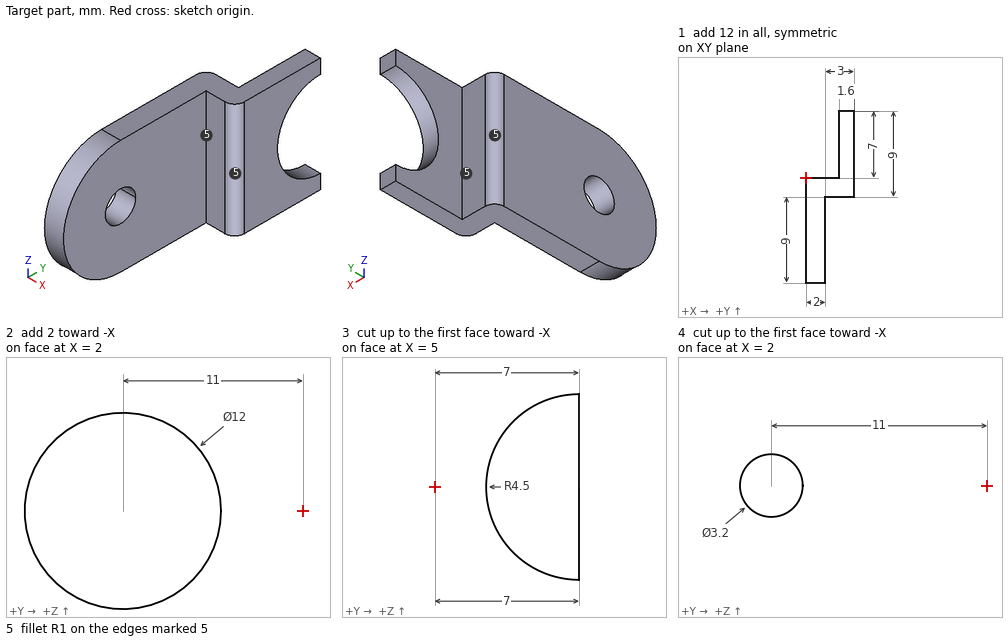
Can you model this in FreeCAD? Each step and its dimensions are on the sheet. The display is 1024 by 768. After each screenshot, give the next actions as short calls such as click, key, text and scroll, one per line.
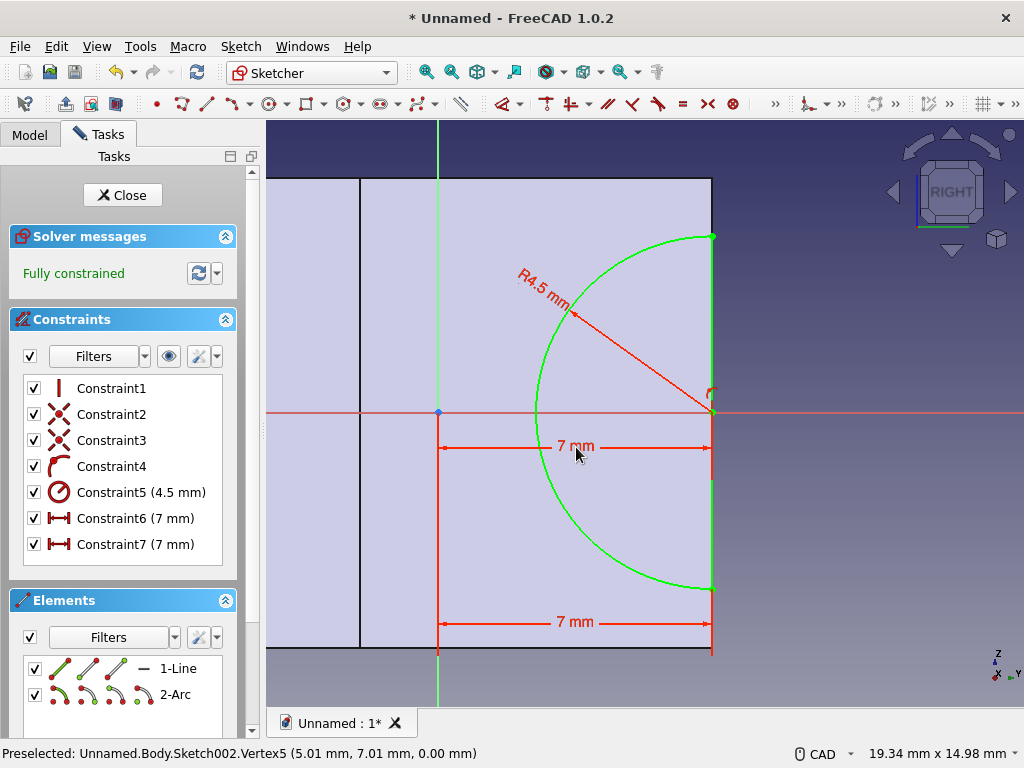
click(123, 195)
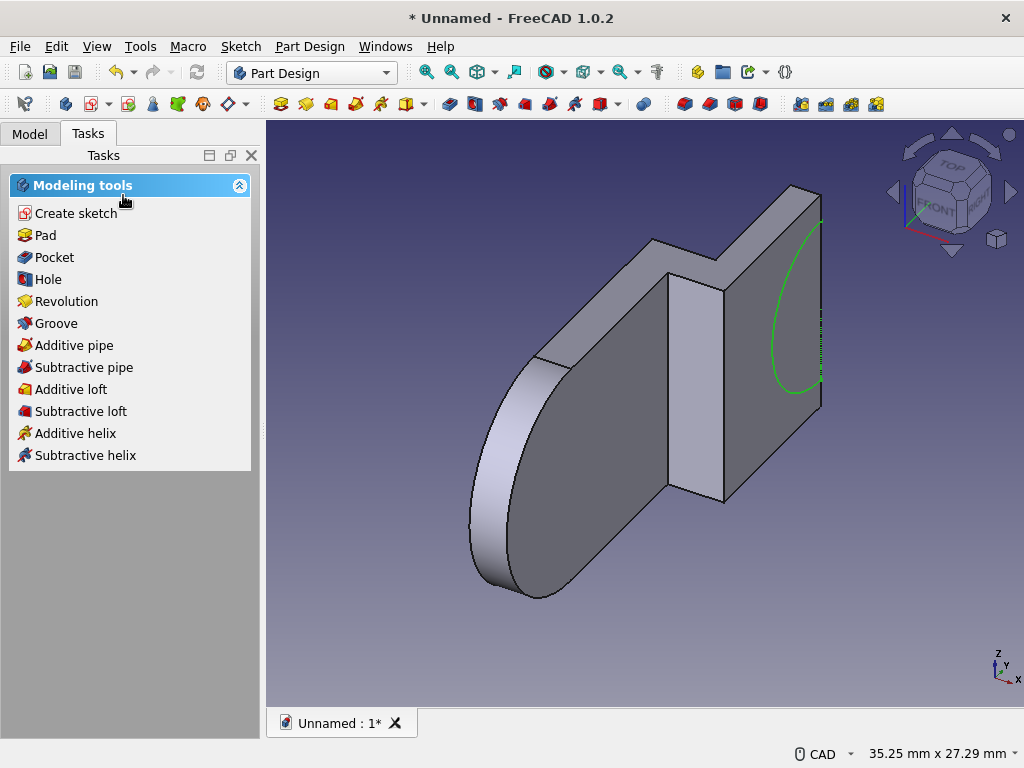
click(450, 104)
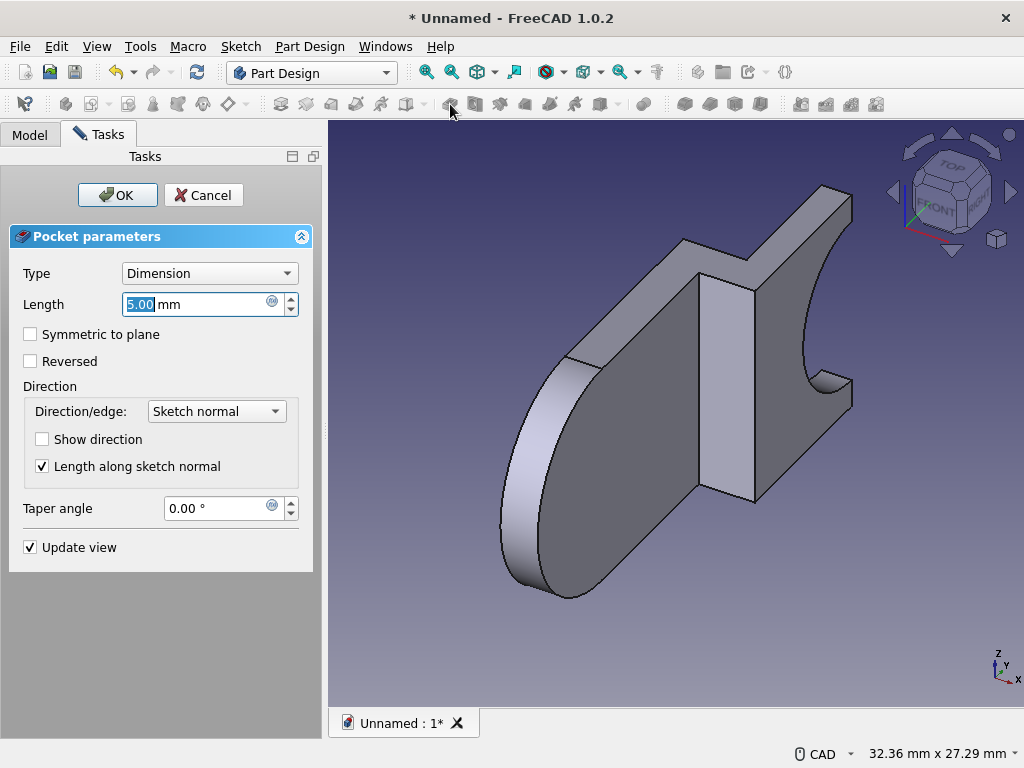
click(210, 274)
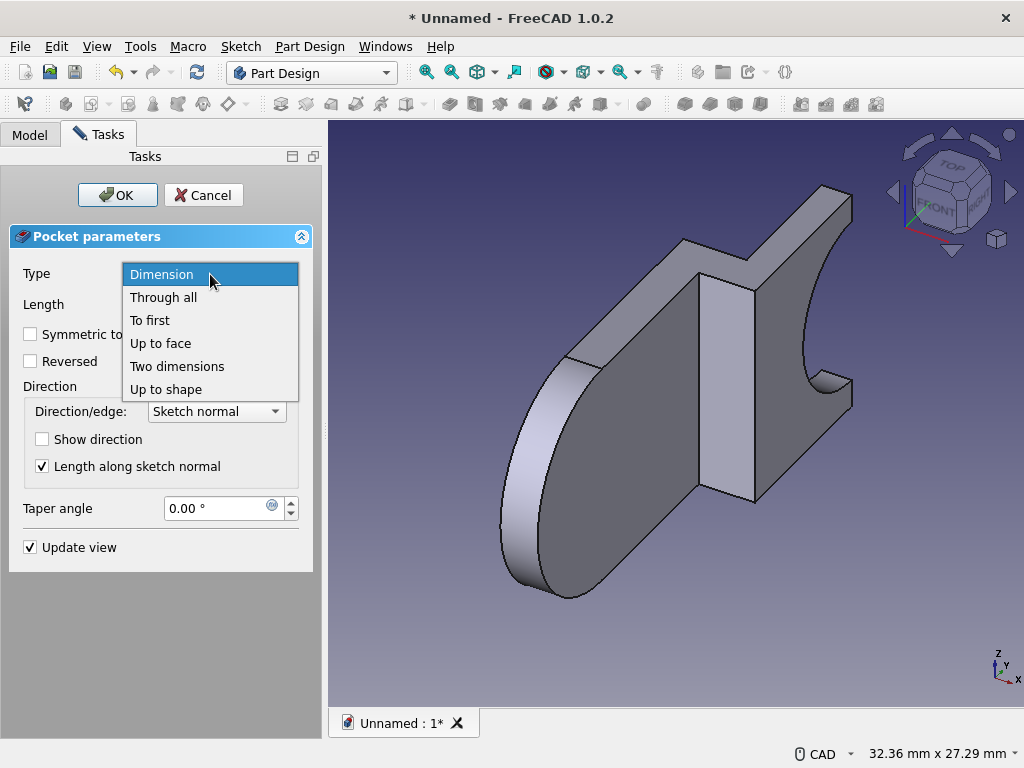
click(208, 320)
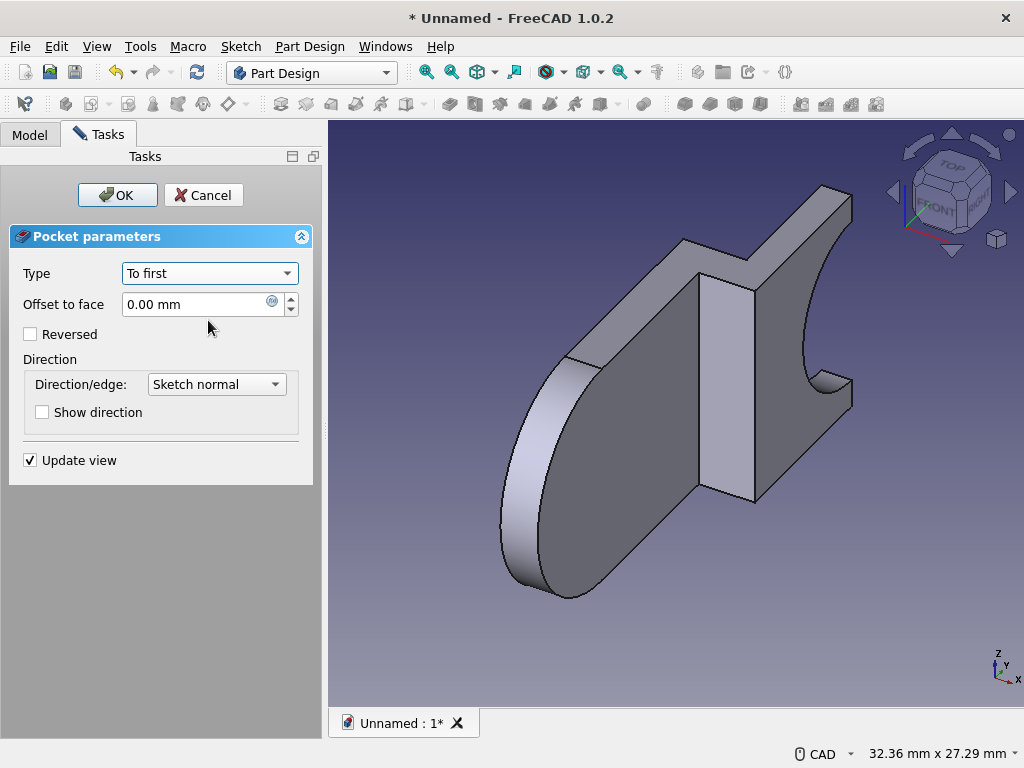
click(118, 195)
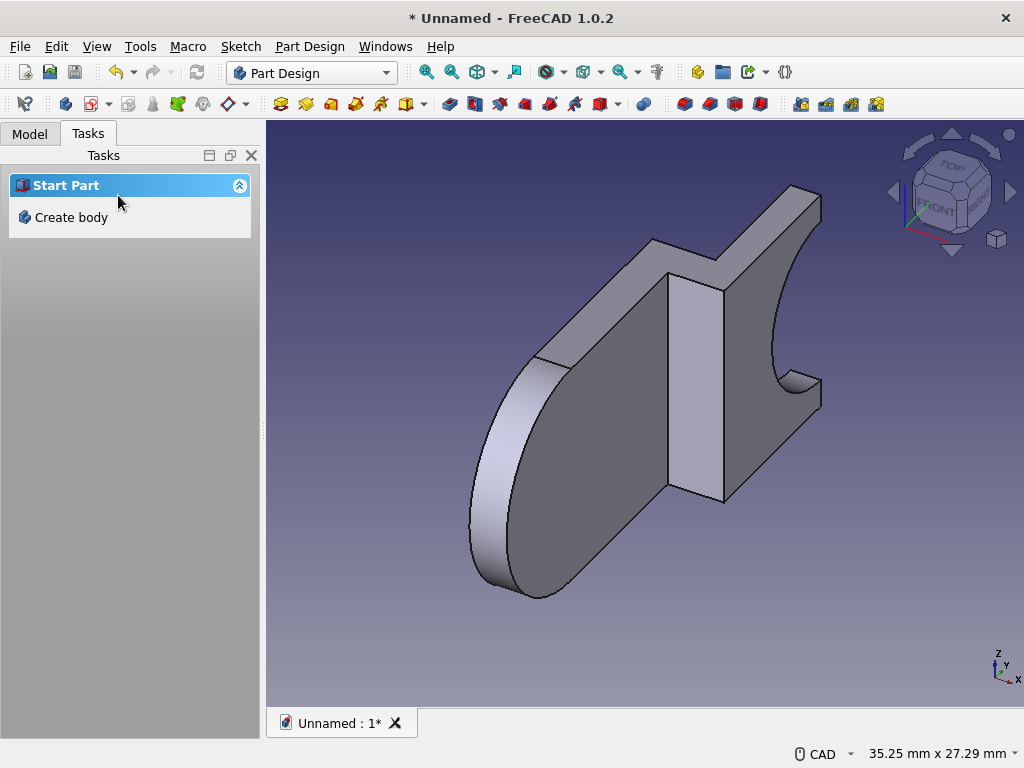
click(587, 457)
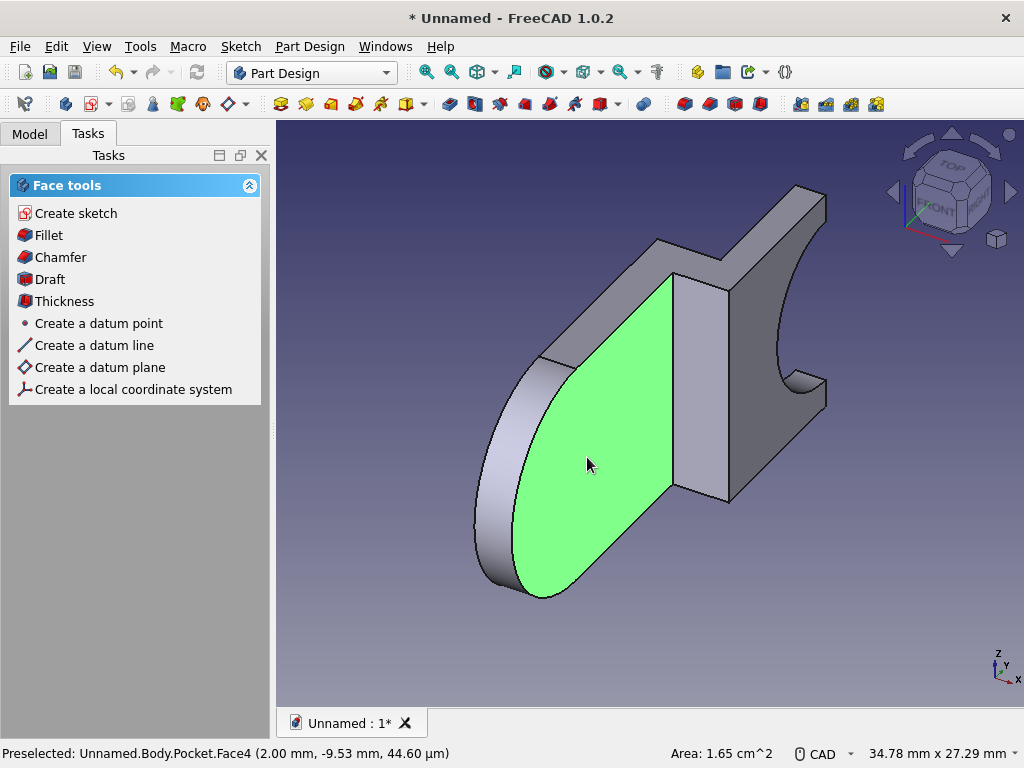
click(90, 104)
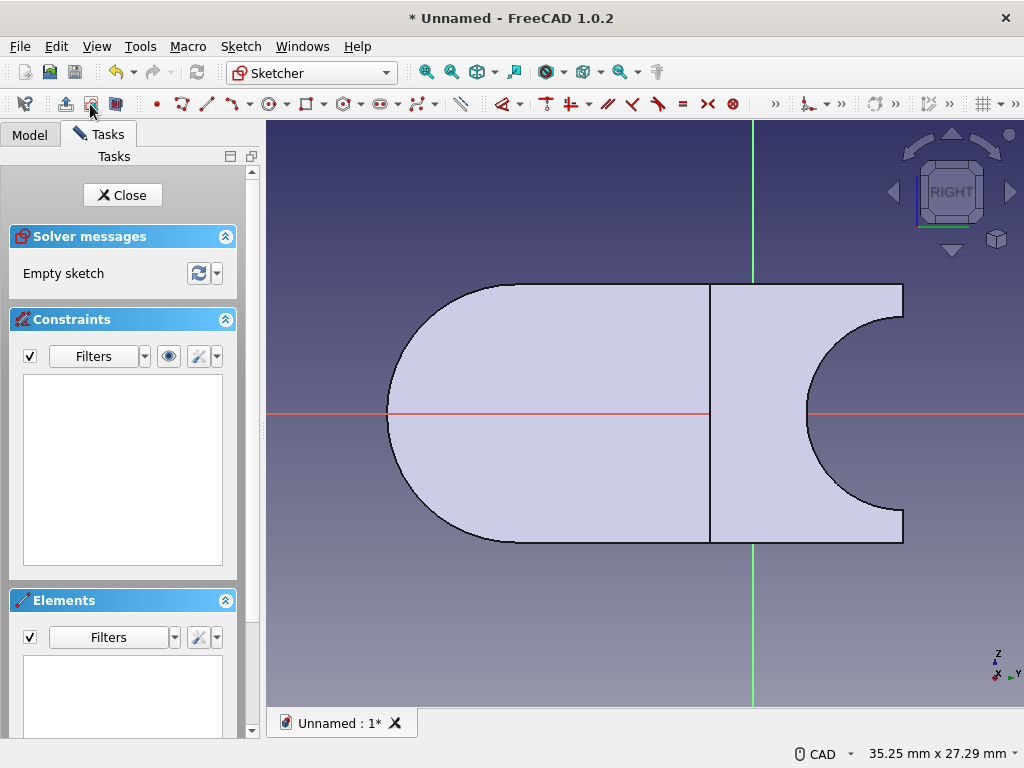
key(q)
key(s)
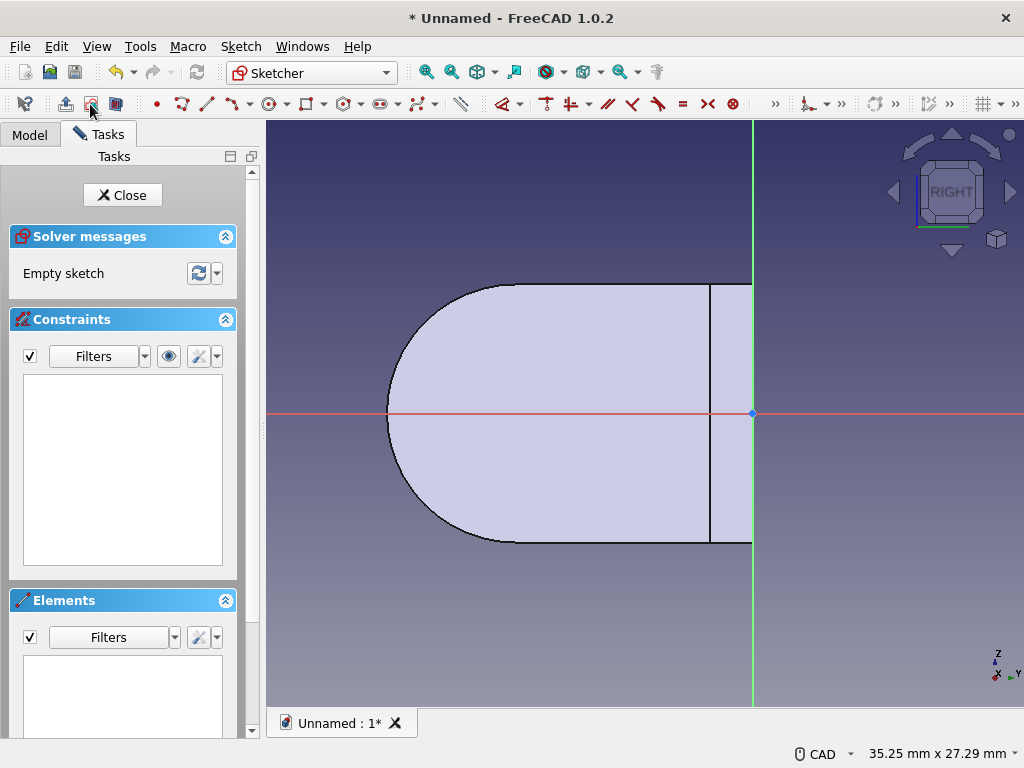
scroll(501, 414, up, 8)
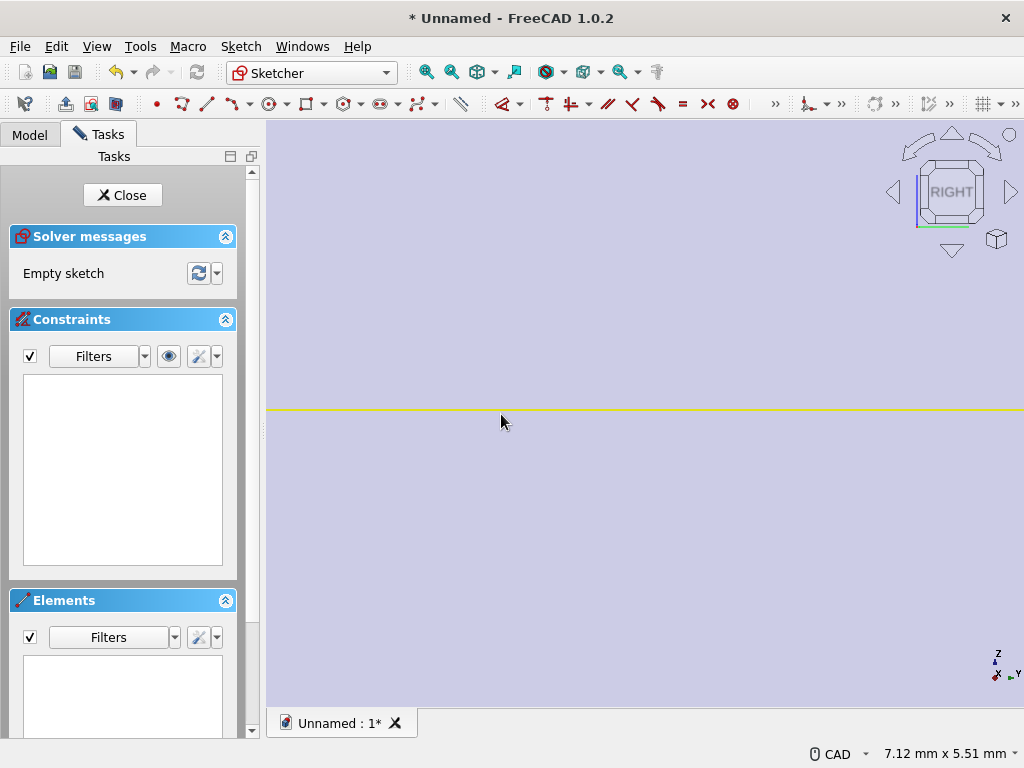
key(g)
key(c)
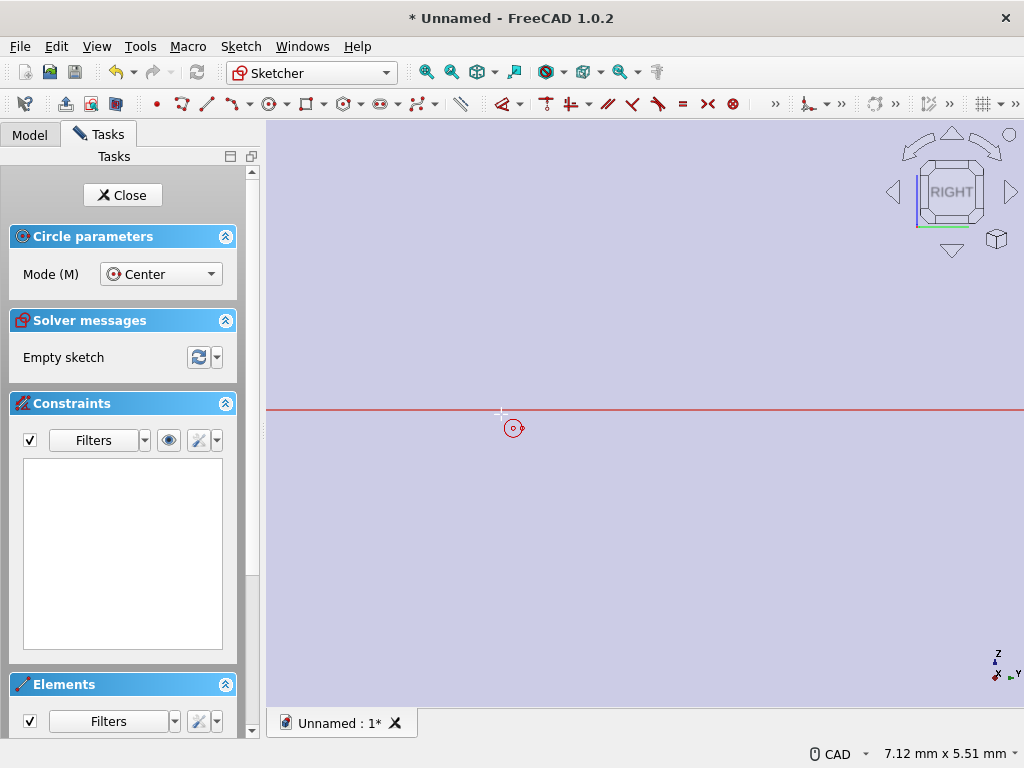
click(574, 410)
move(694, 289)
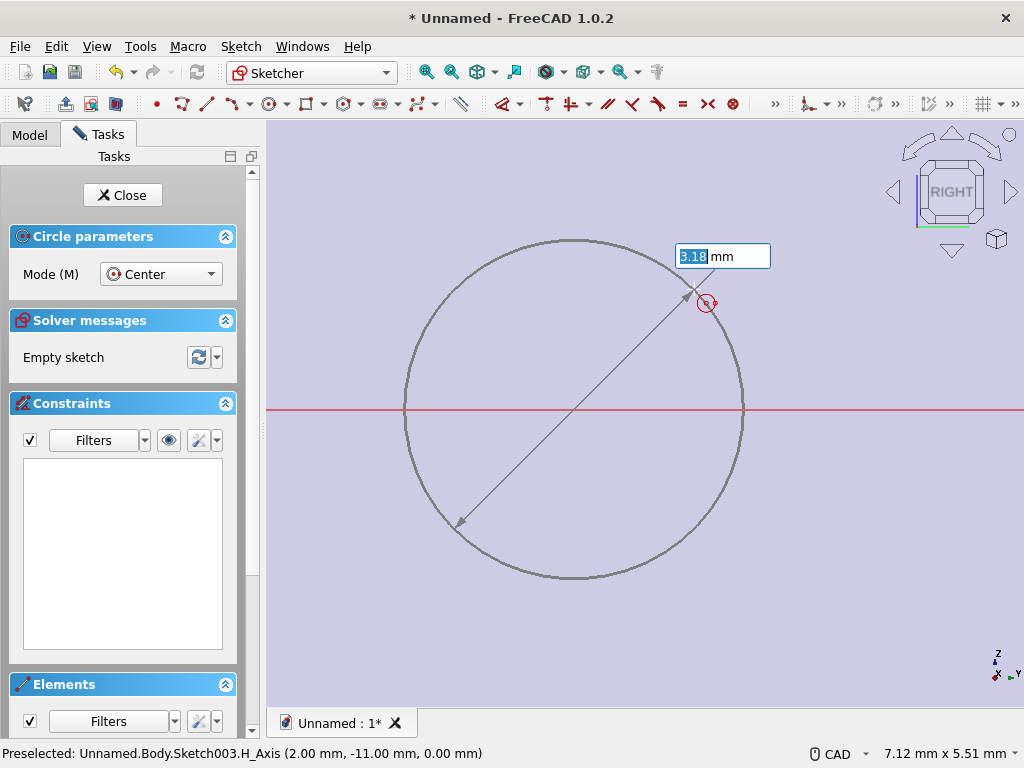
text(3.2)
key(Return)
key(Escape)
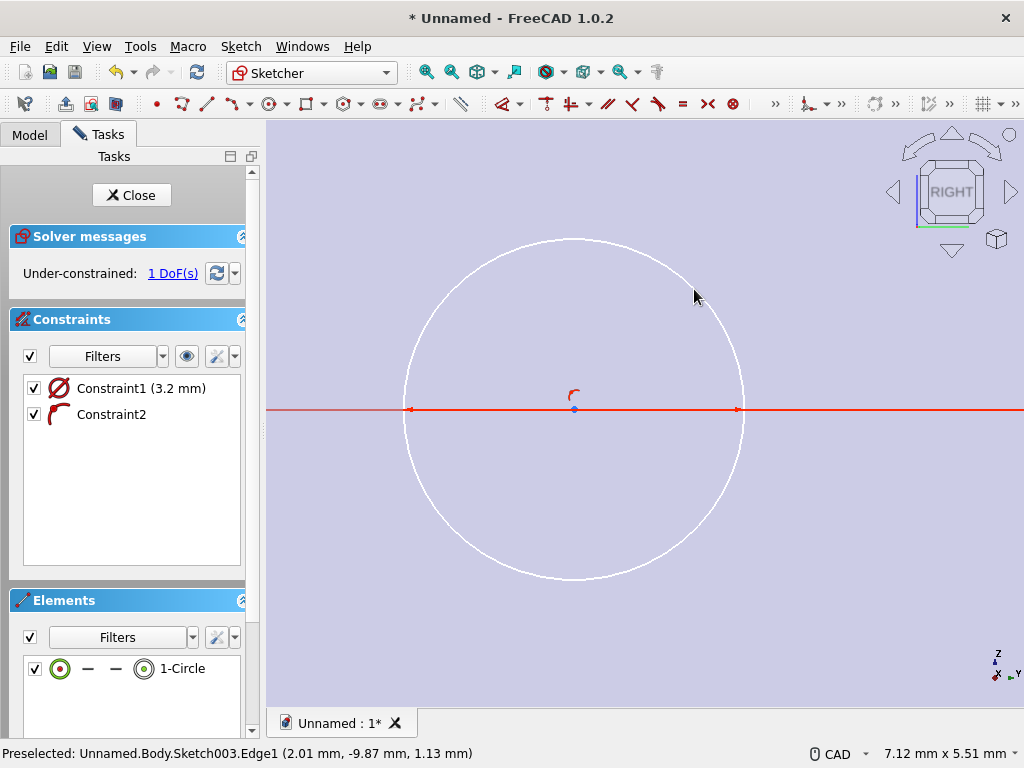
key(d)